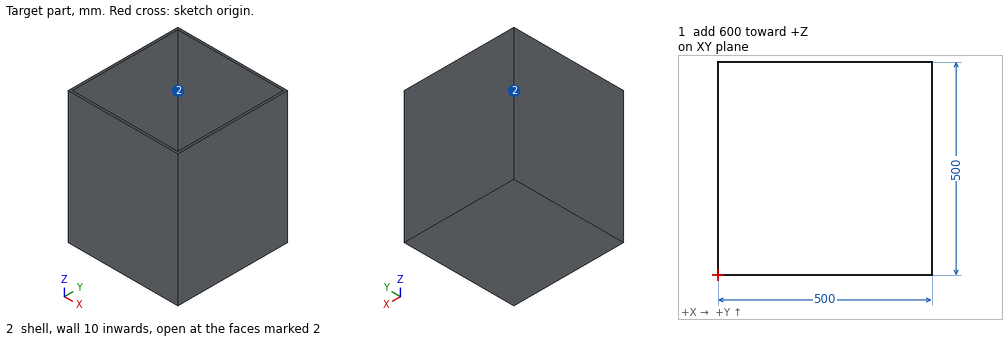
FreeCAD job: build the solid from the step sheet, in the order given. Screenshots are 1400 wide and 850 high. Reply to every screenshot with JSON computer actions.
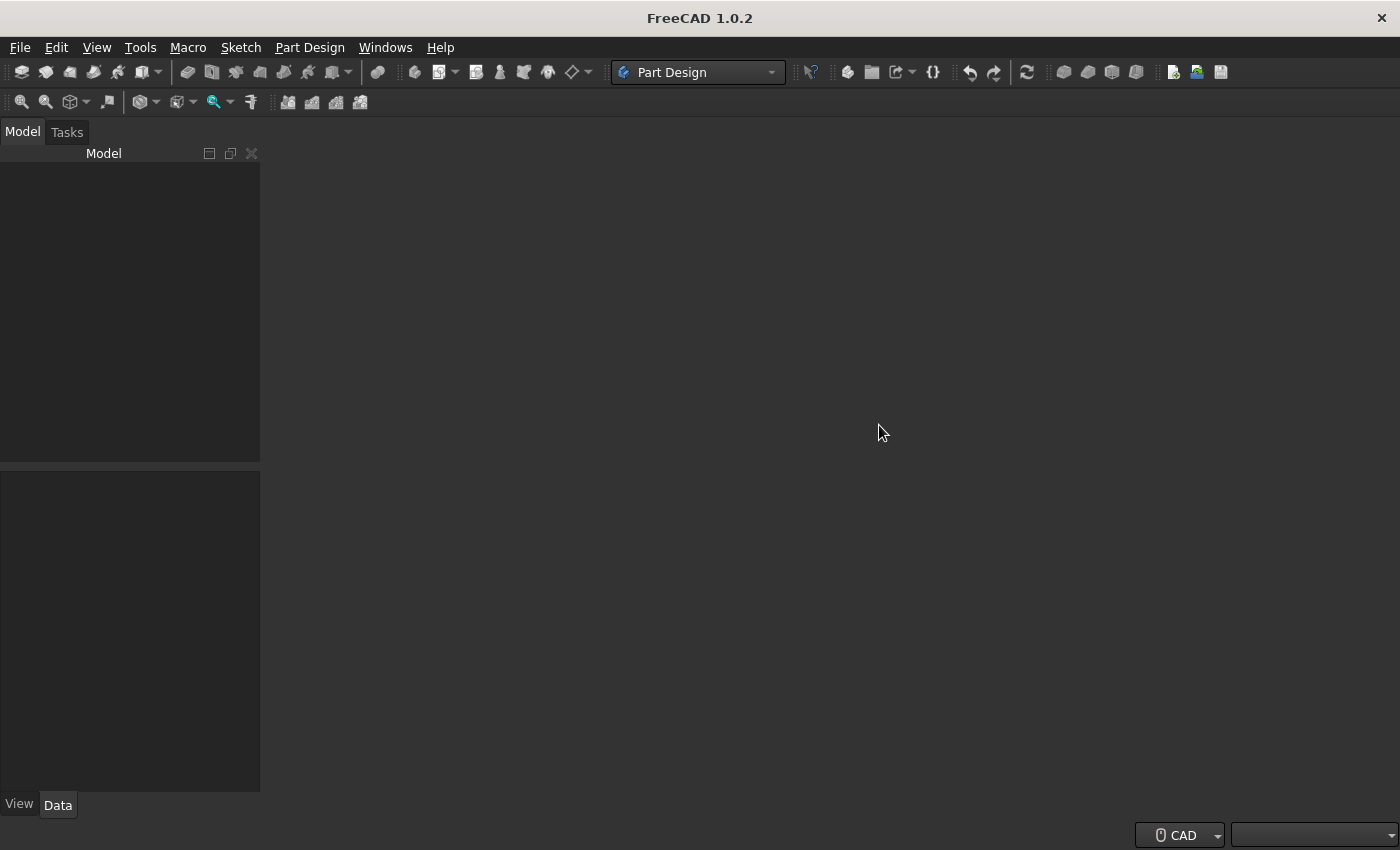
{"action": "left_click", "coordinate": [1174, 72]}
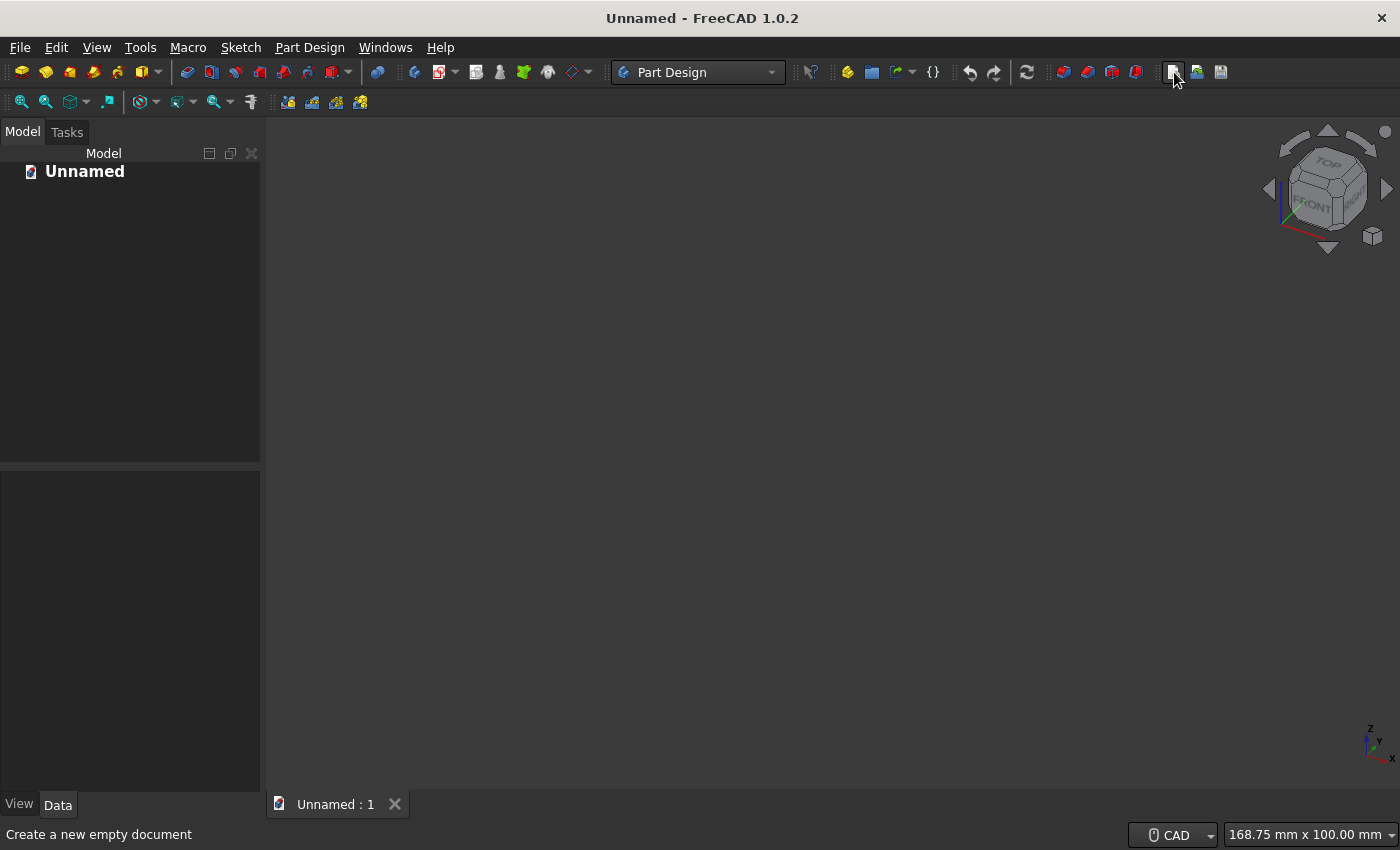
{"action": "left_click", "coordinate": [440, 72]}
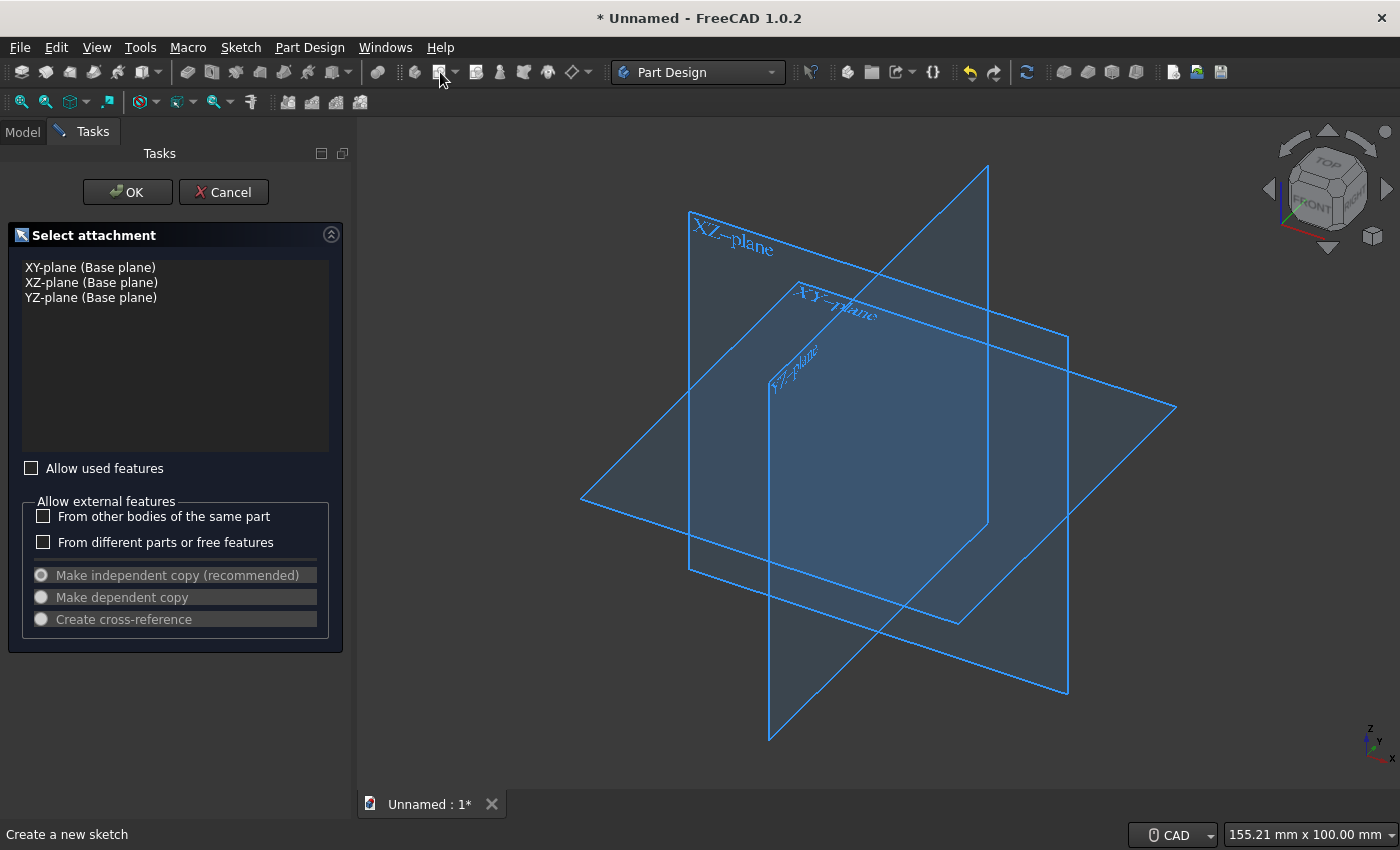
{"action": "left_click", "coordinate": [82, 268]}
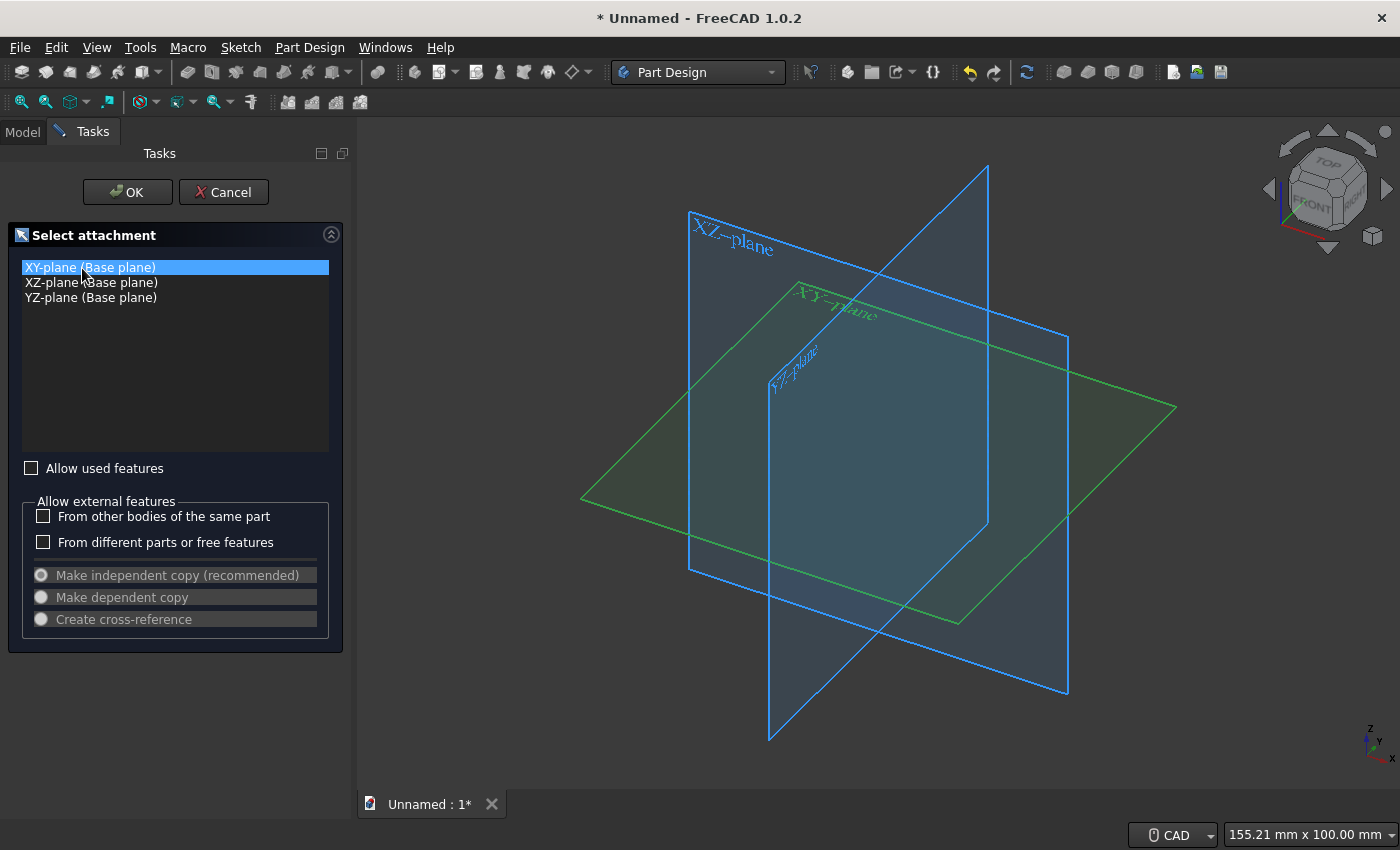
{"action": "left_click", "coordinate": [128, 192]}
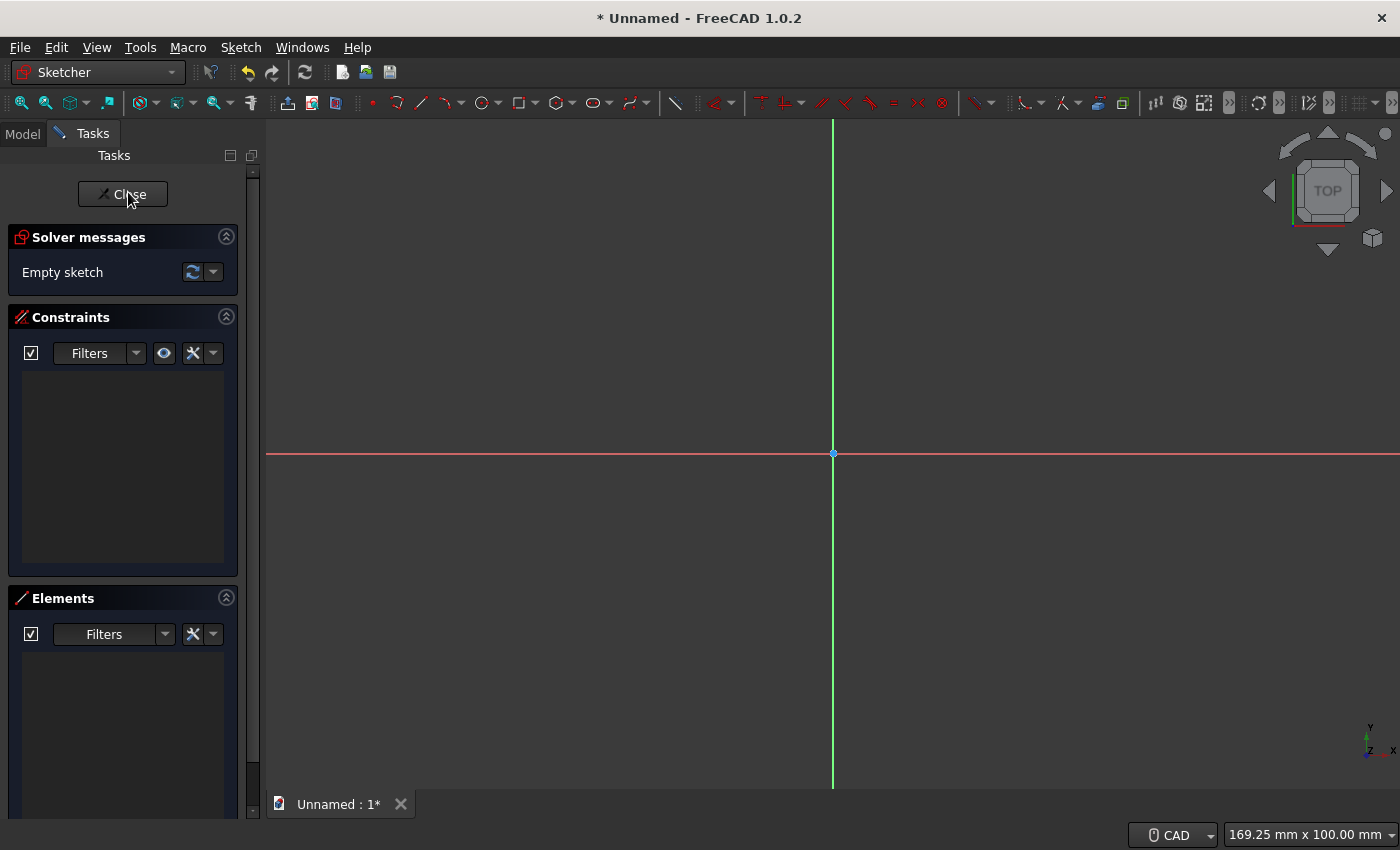
{"action": "scroll", "coordinate": [492, 716], "scroll_direction": "down", "scroll_amount": 10}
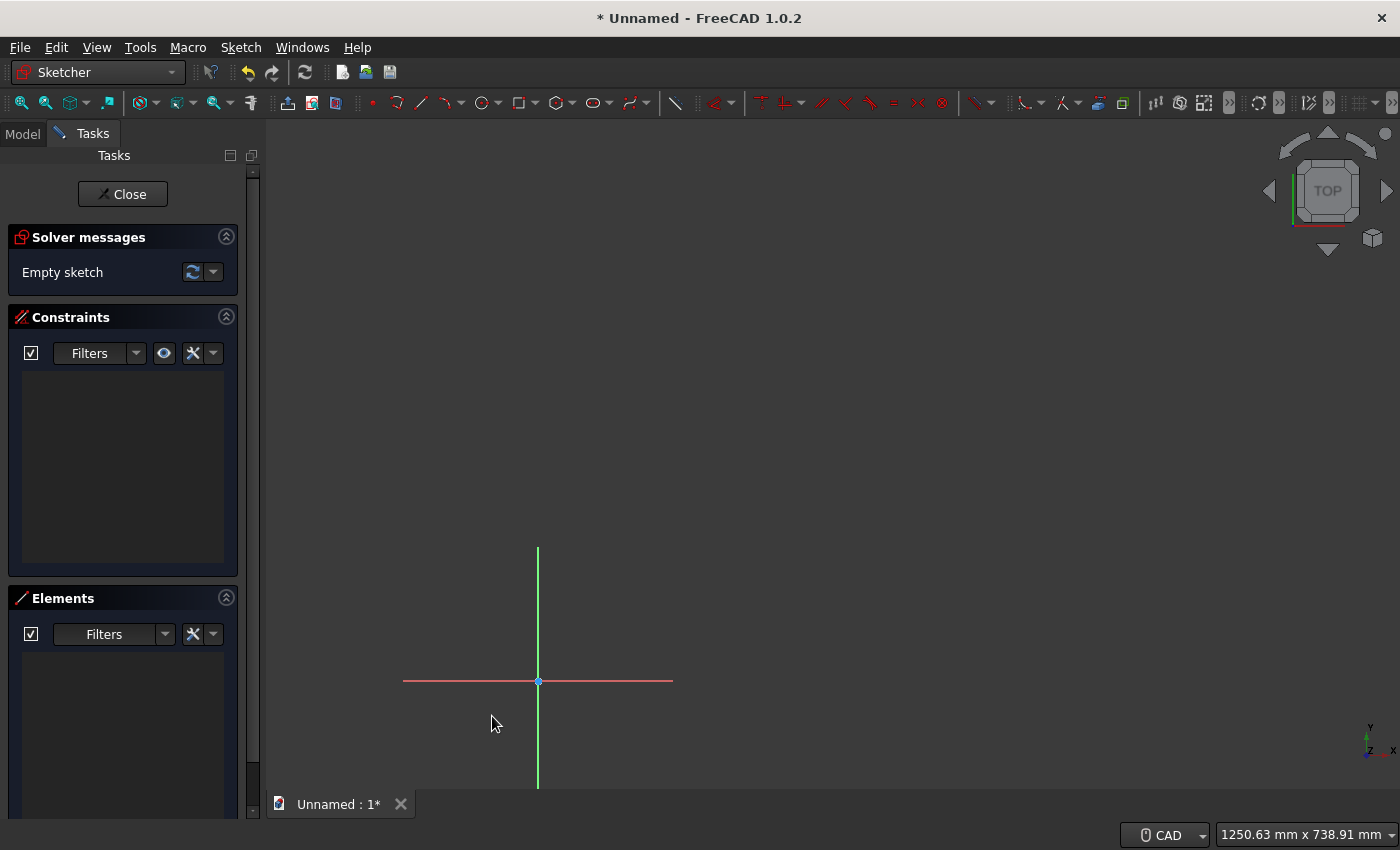
{"action": "left_click", "coordinate": [520, 104]}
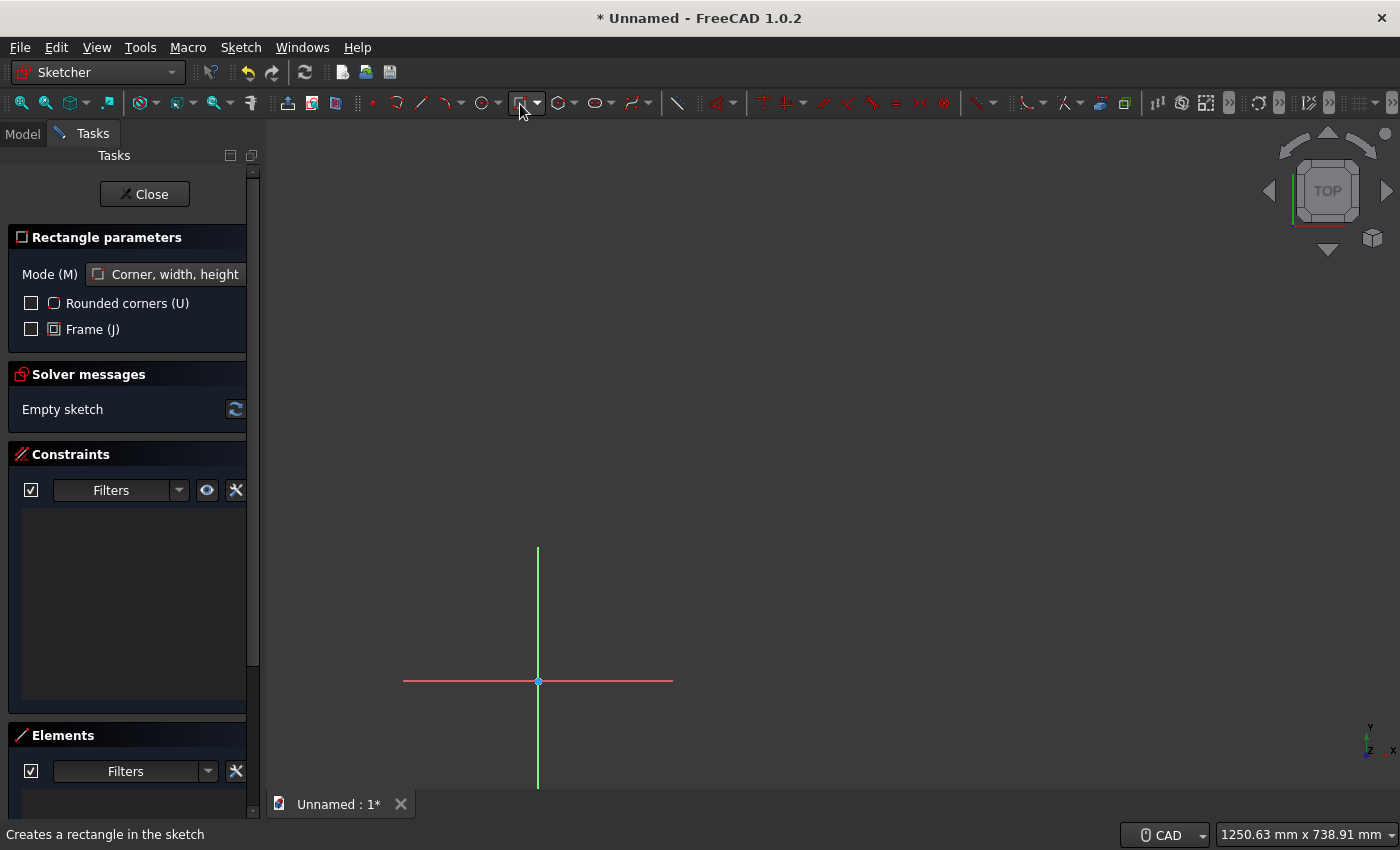
{"action": "left_click", "coordinate": [538, 681]}
{"action": "left_click", "coordinate": [992, 228]}
{"action": "key", "text": "Escape"}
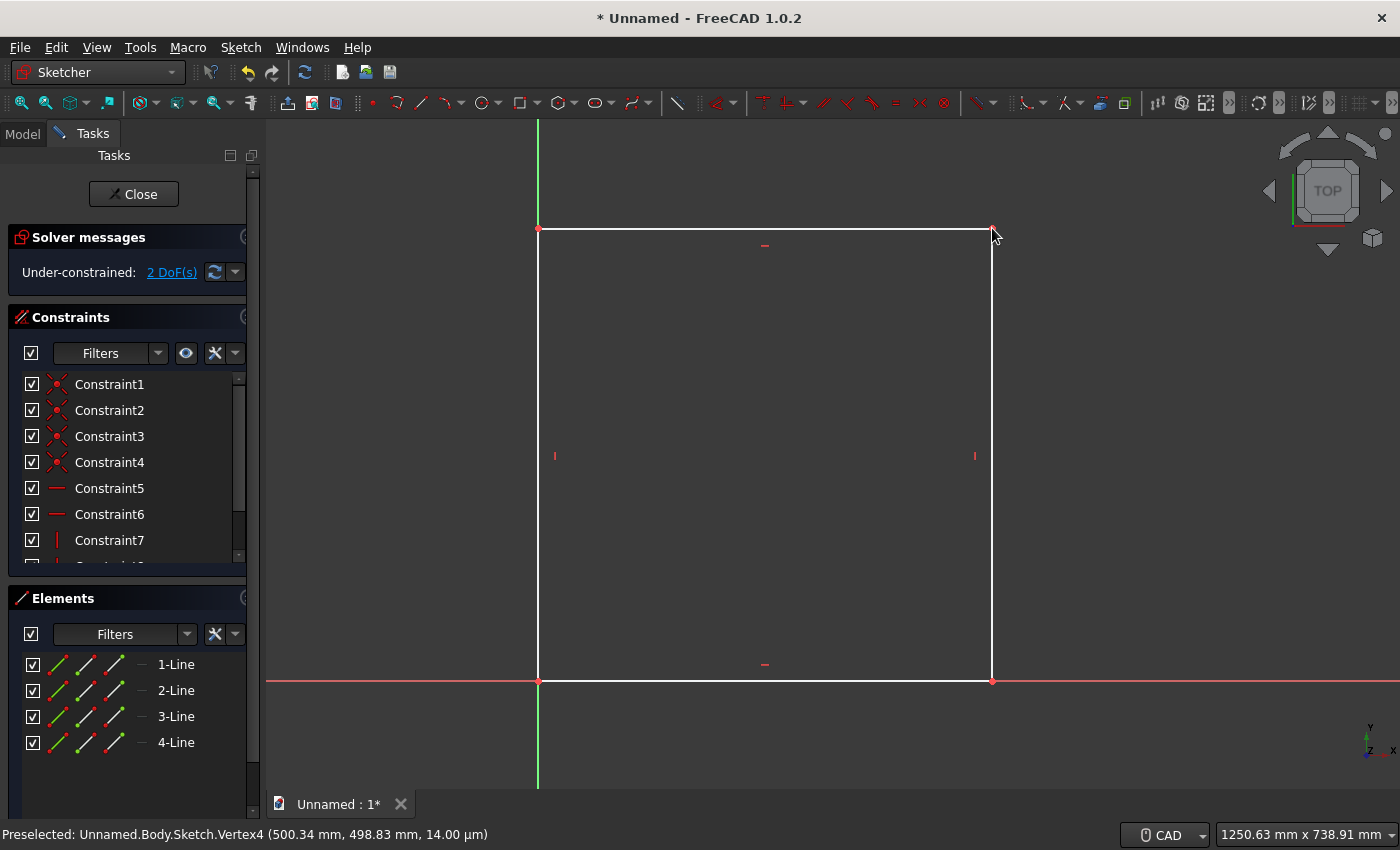
{"action": "key", "text": "d"}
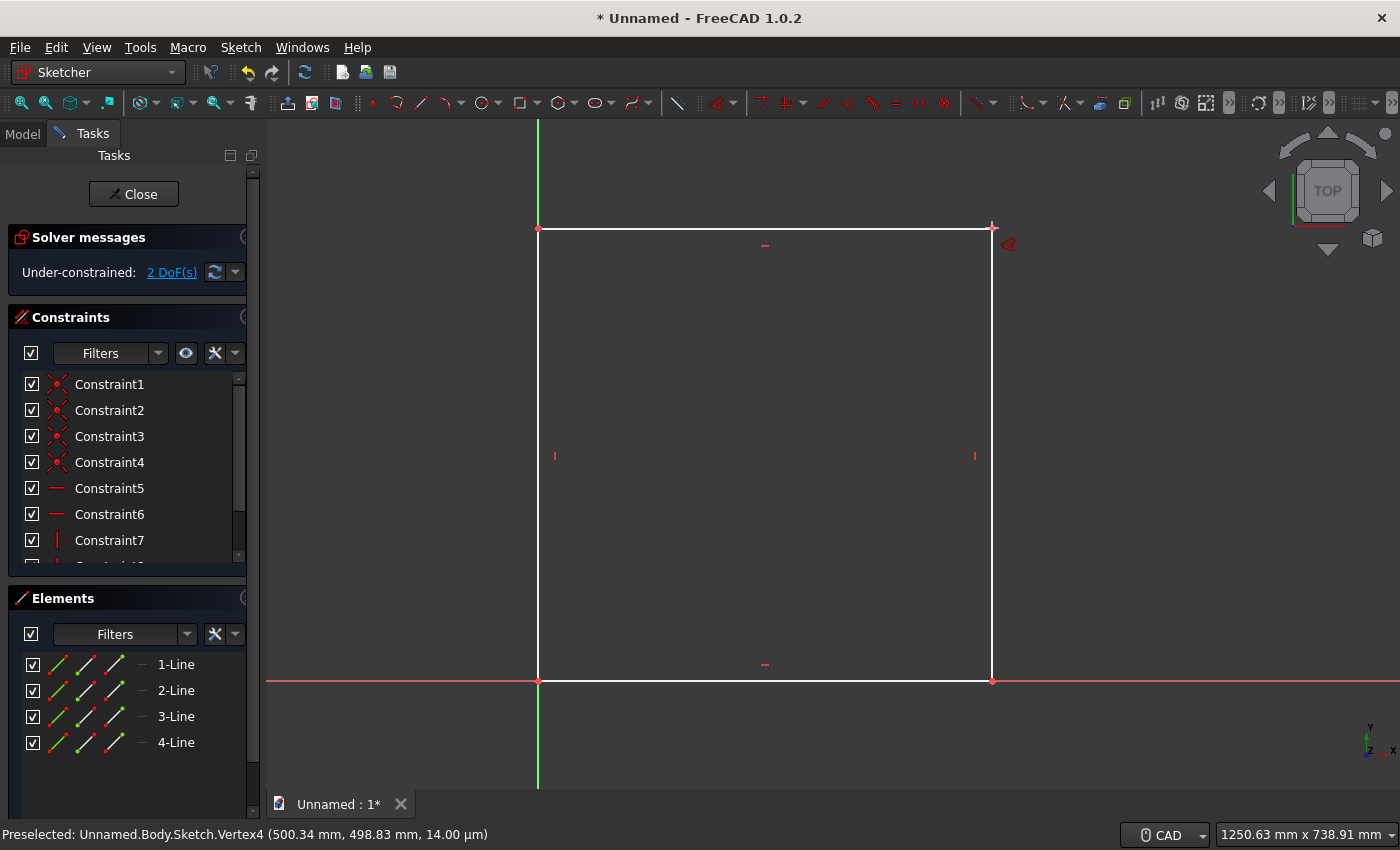
{"action": "left_click", "coordinate": [674, 681]}
{"action": "left_click", "coordinate": [765, 715]}